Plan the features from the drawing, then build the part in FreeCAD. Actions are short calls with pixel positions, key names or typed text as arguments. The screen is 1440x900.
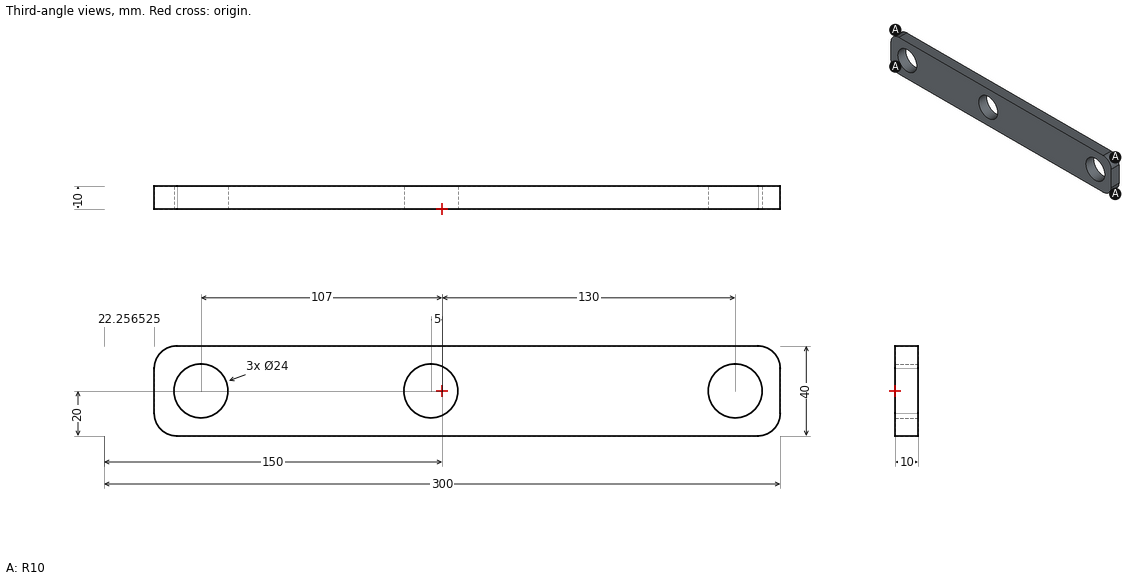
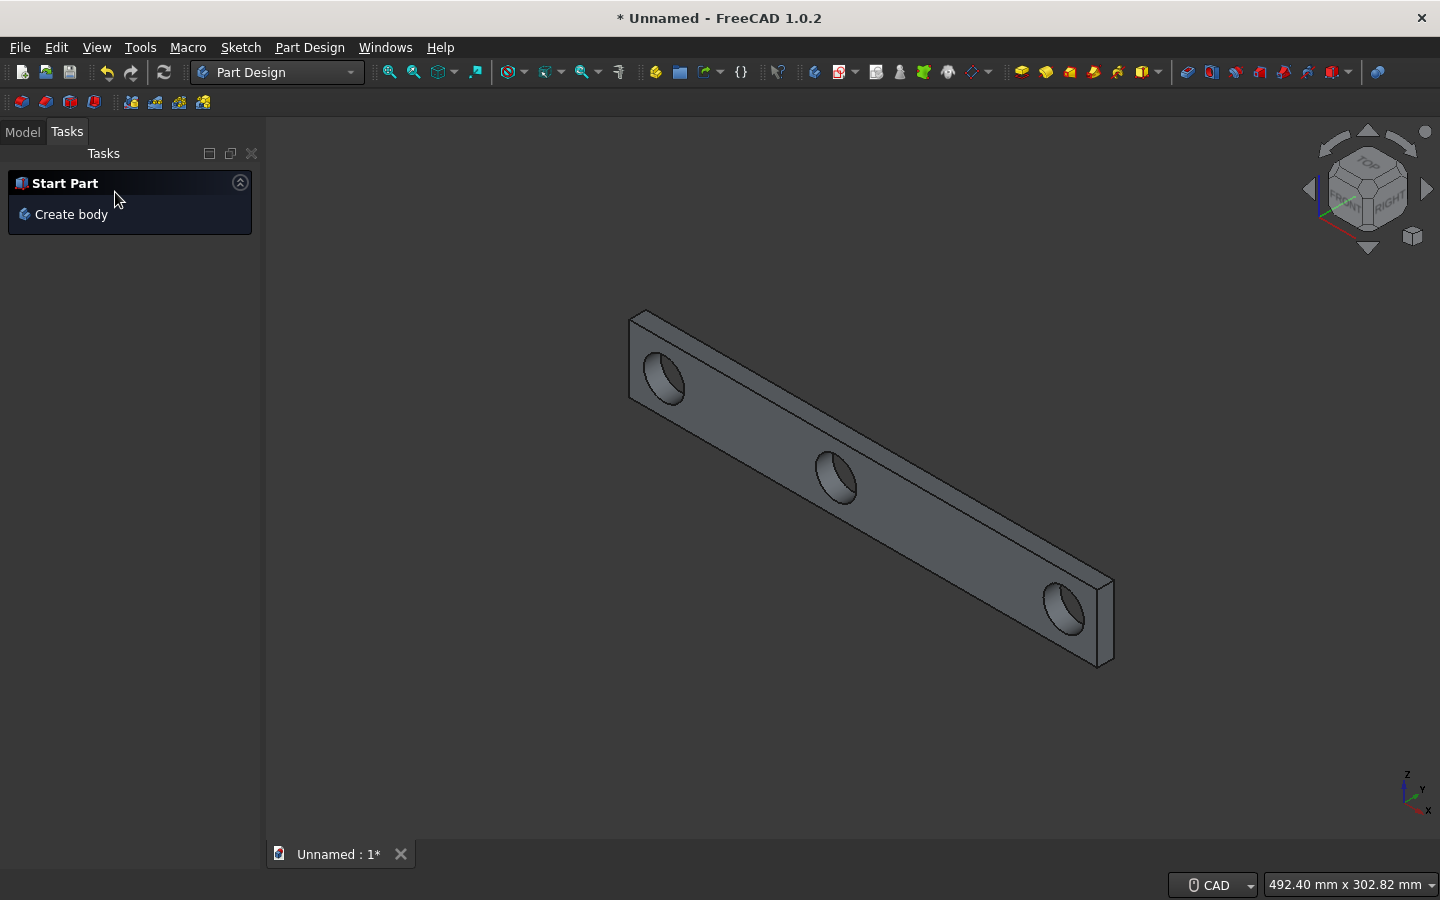
click(1106, 584)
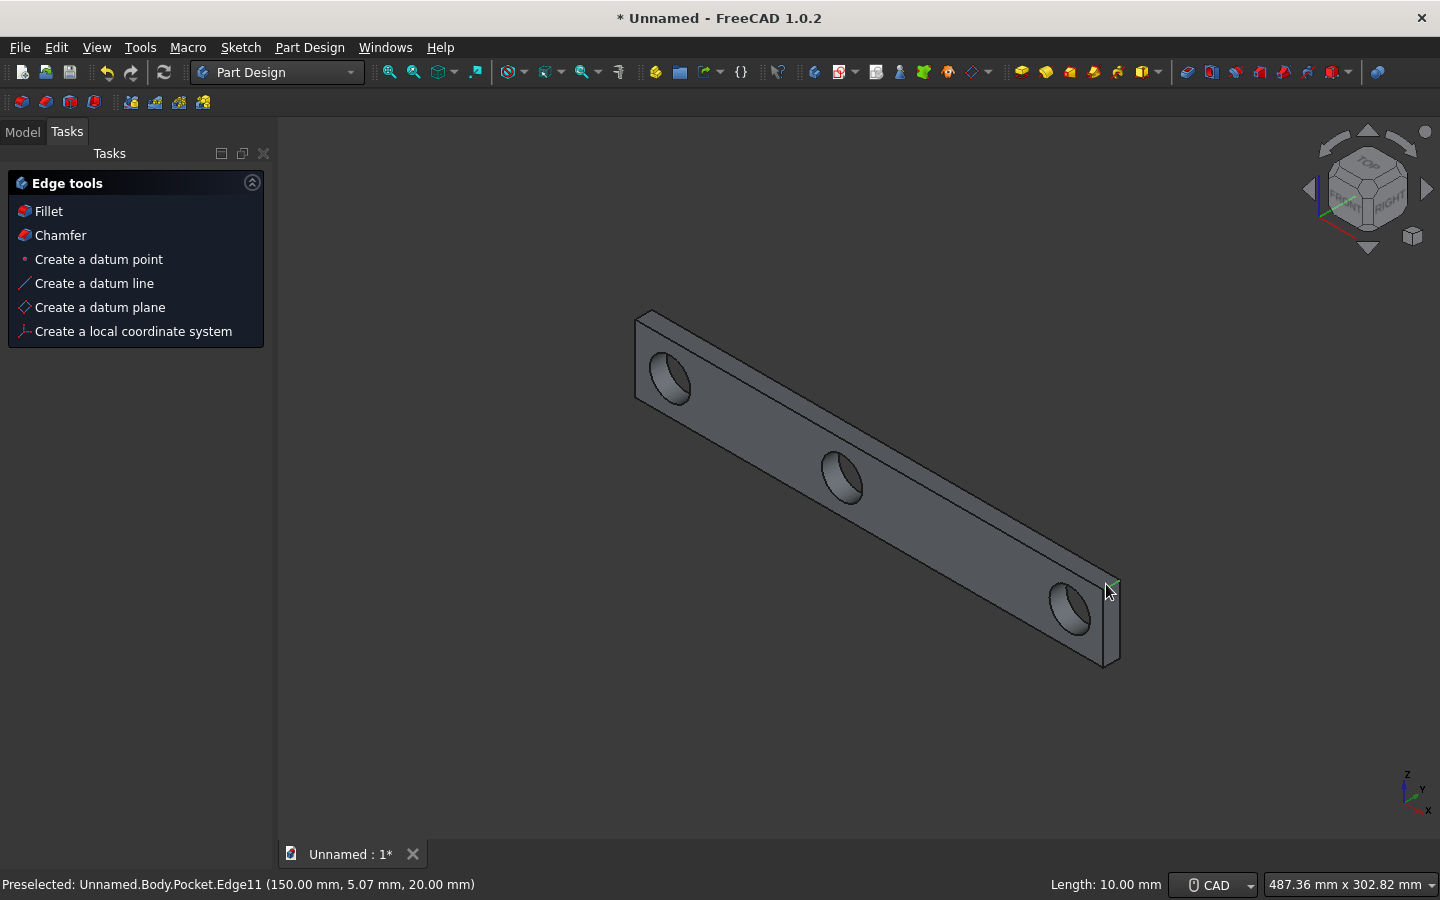
key(2)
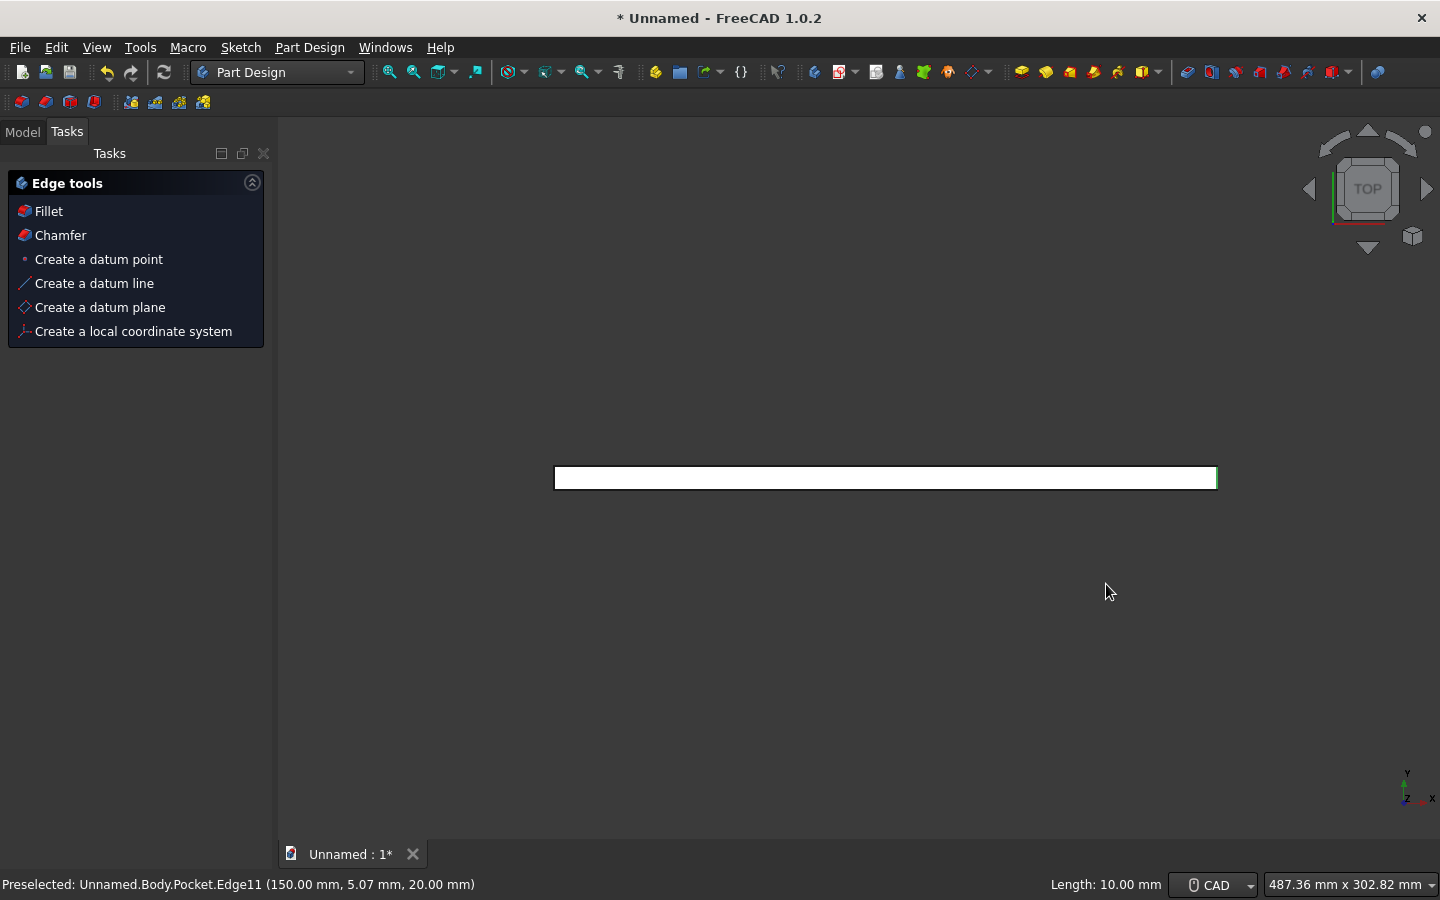
click(554, 477, ctrl)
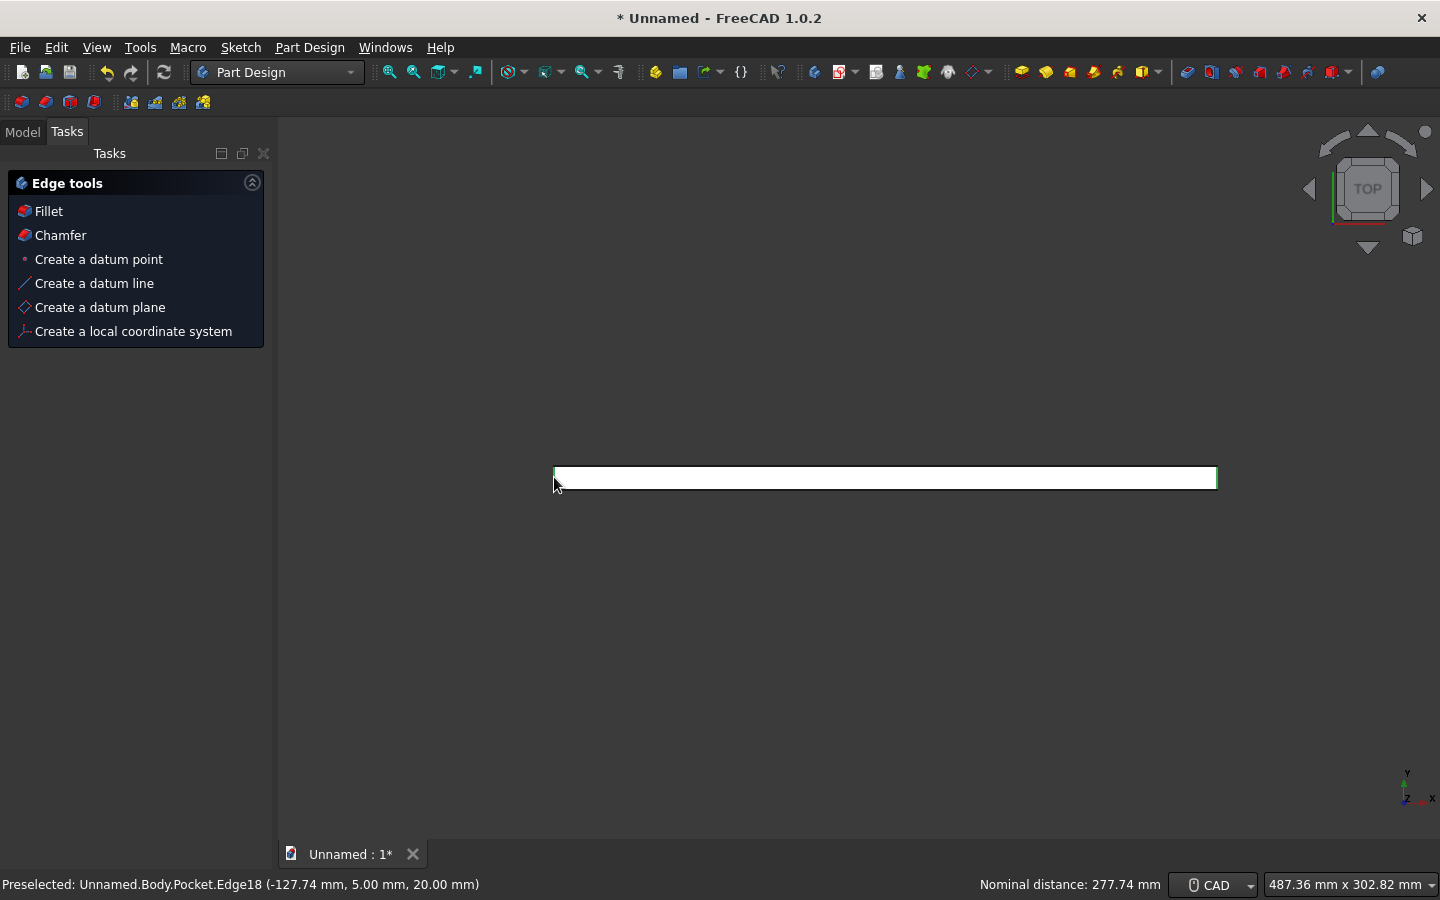
key(1)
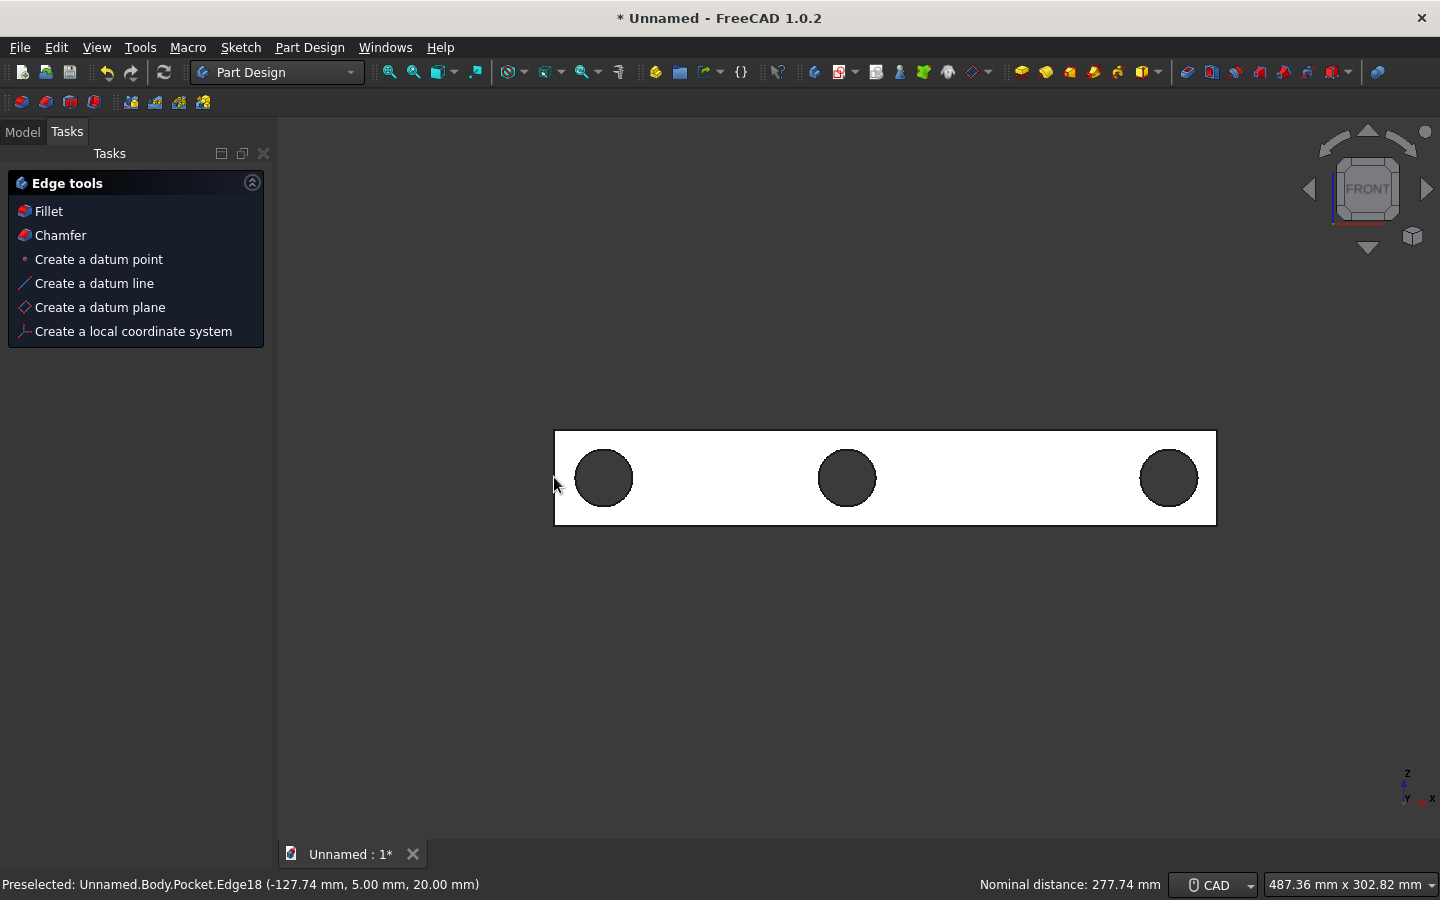
key(3)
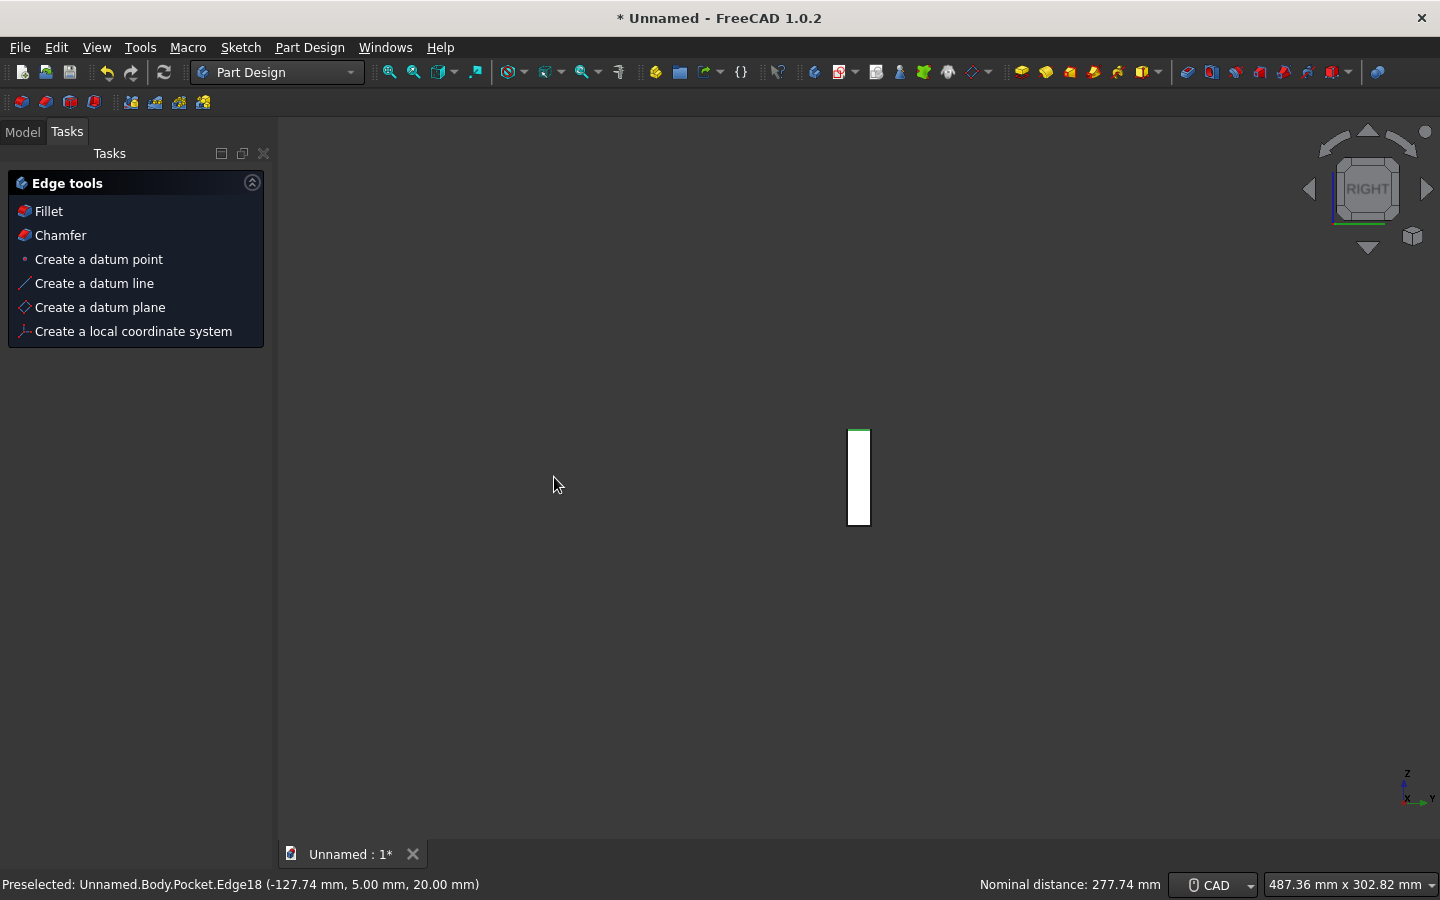
click(390, 72)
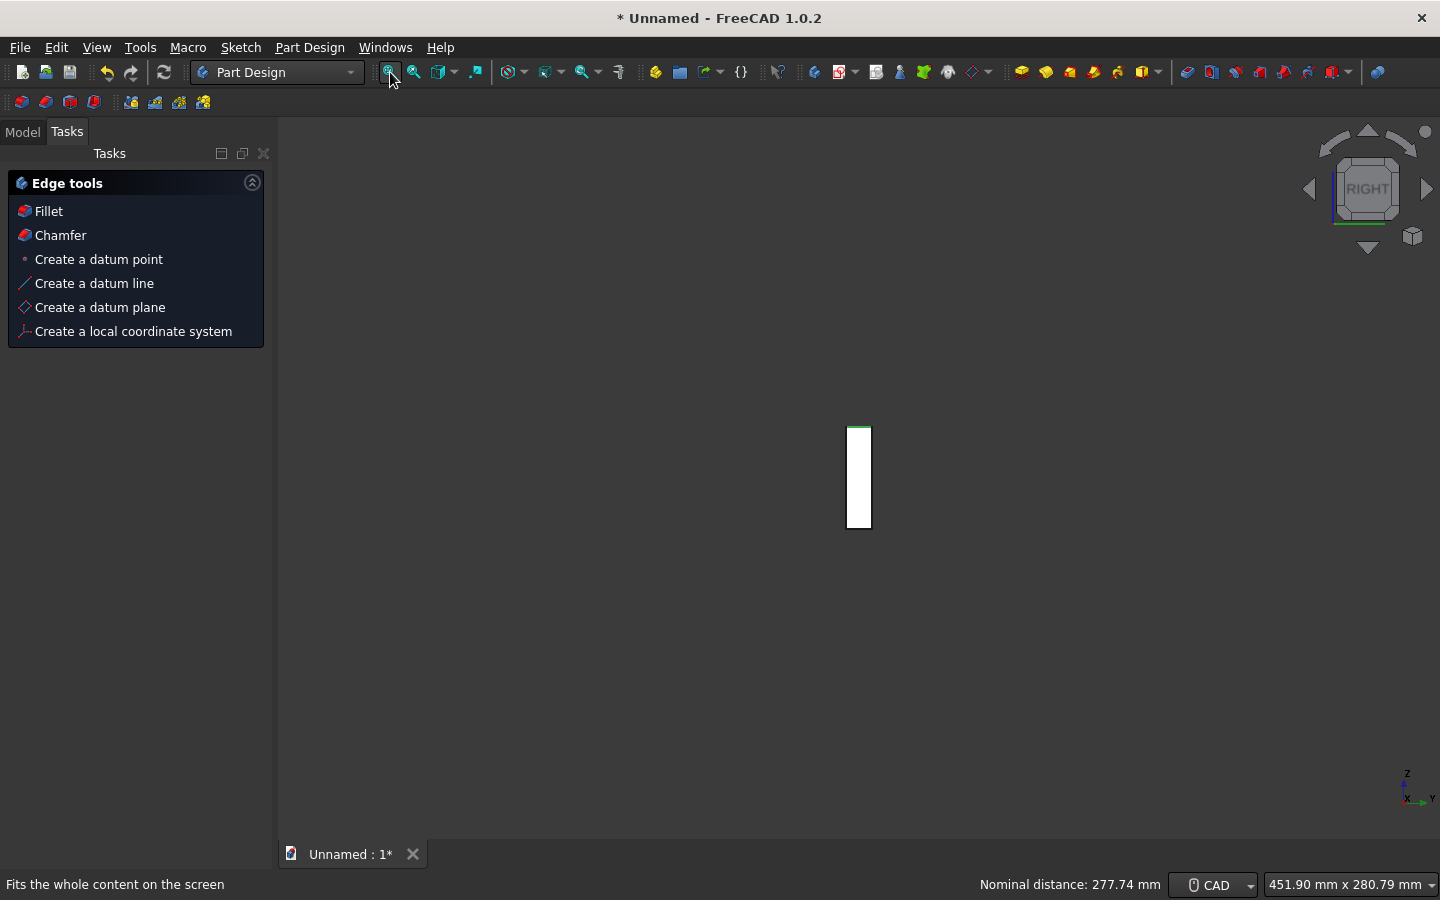
click(859, 528, ctrl)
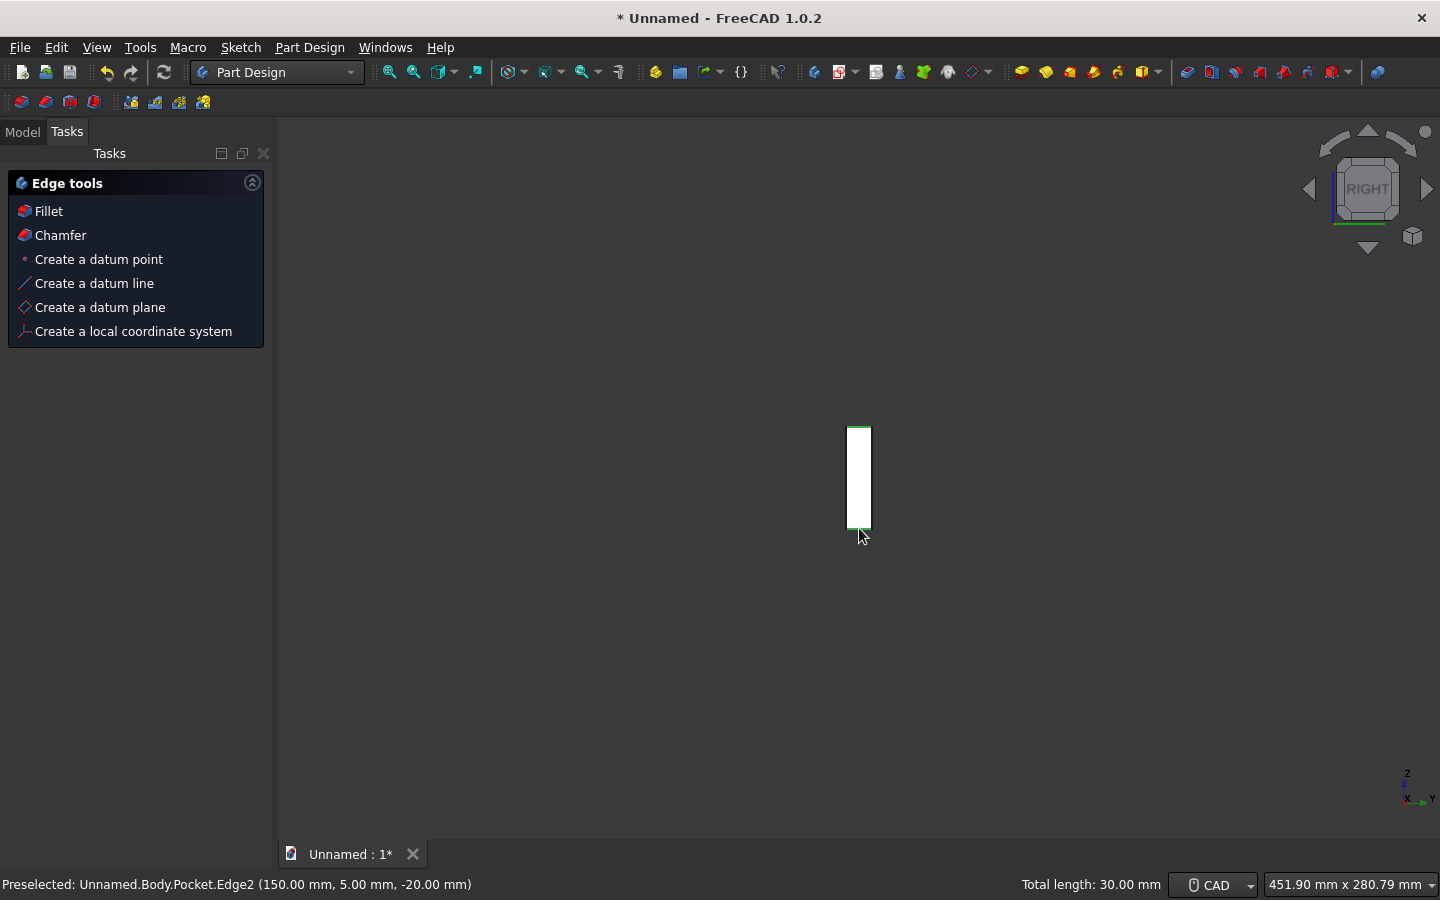
key(5)